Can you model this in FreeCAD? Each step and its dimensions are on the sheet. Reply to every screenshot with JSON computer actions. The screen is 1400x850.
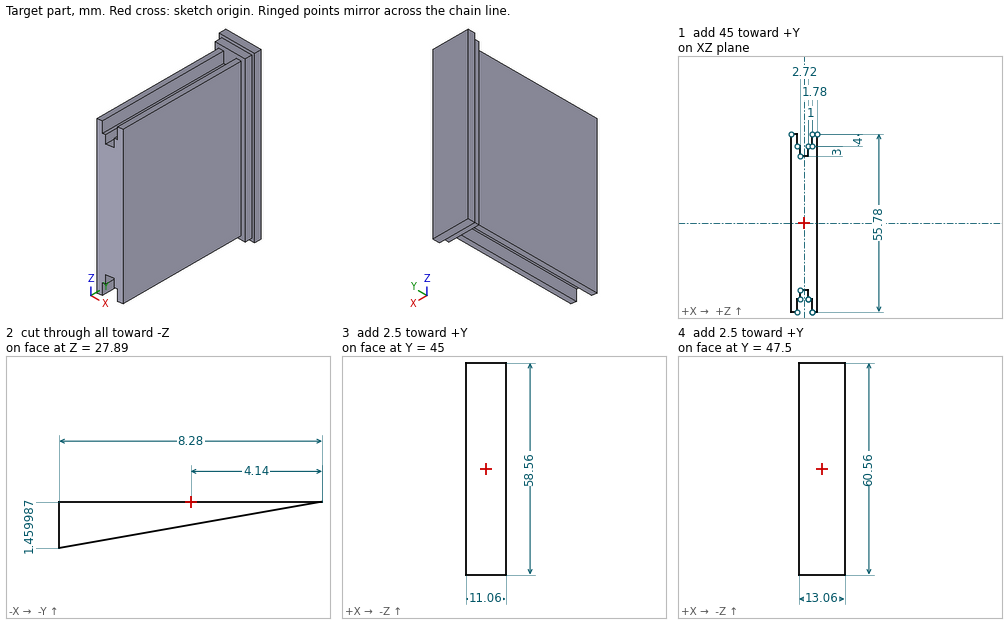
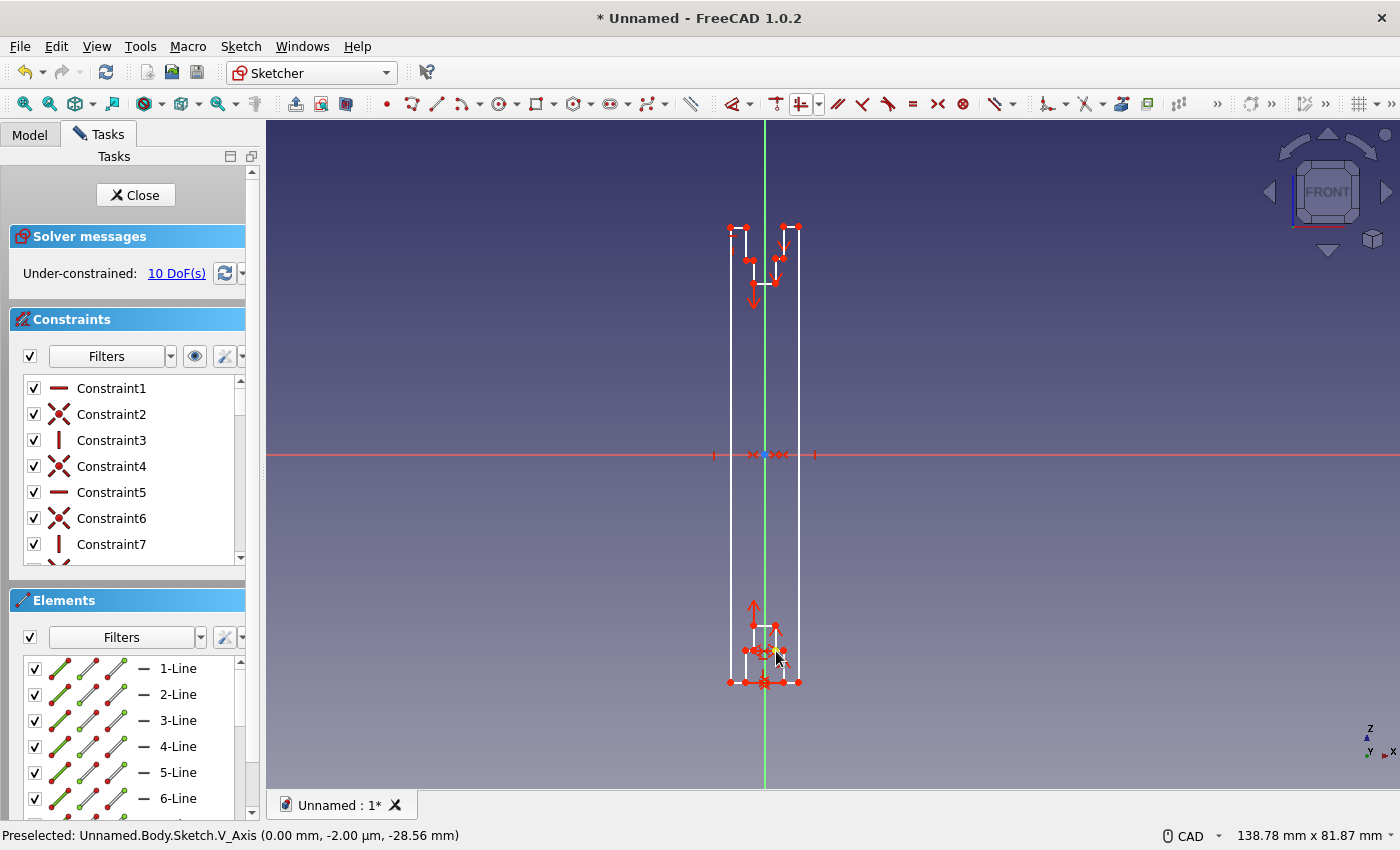
{"action": "left_click", "coordinate": [799, 227]}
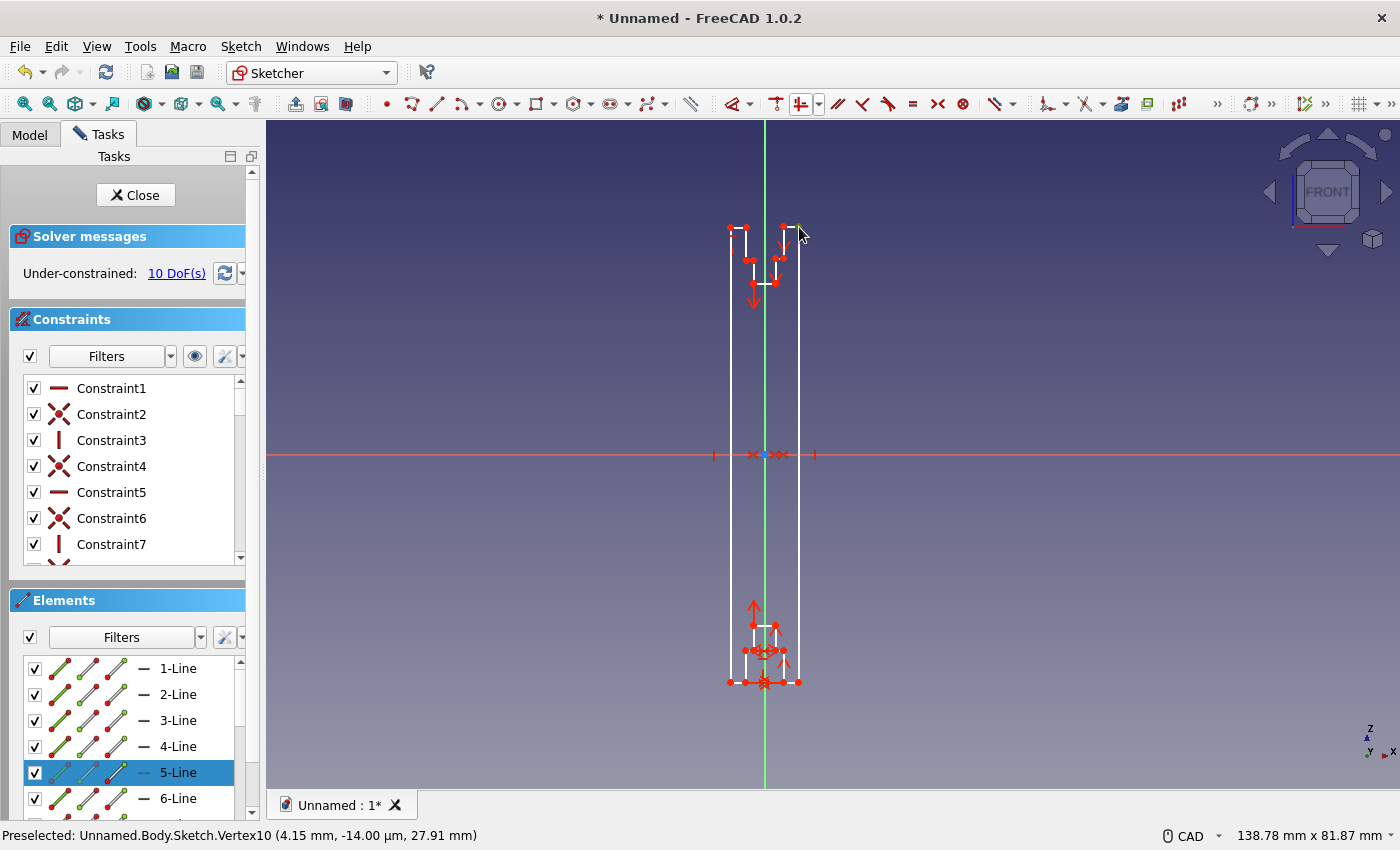
{"action": "left_click", "coordinate": [731, 228]}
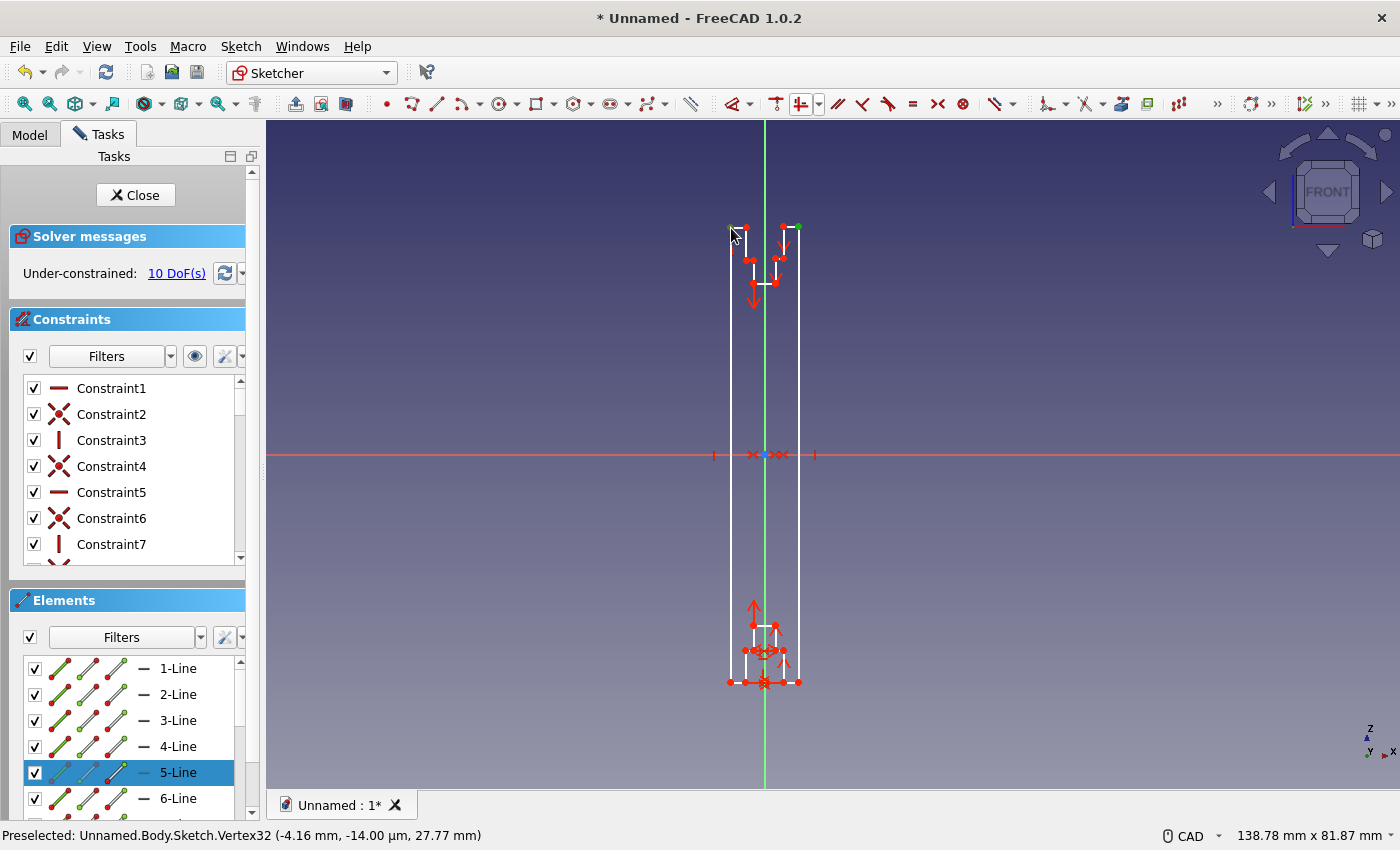
{"action": "left_click", "coordinate": [765, 717]}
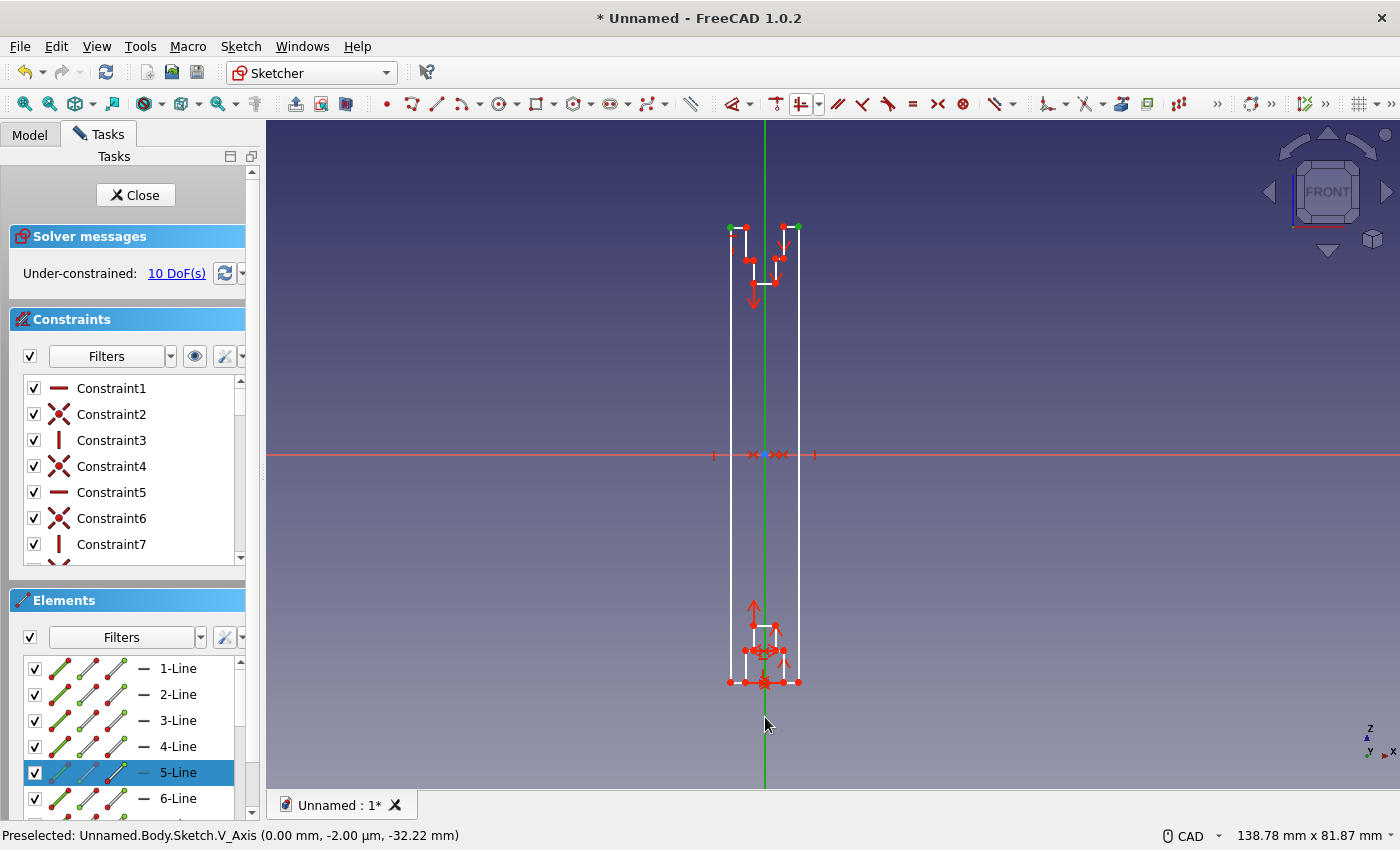
{"action": "left_click", "coordinate": [938, 104]}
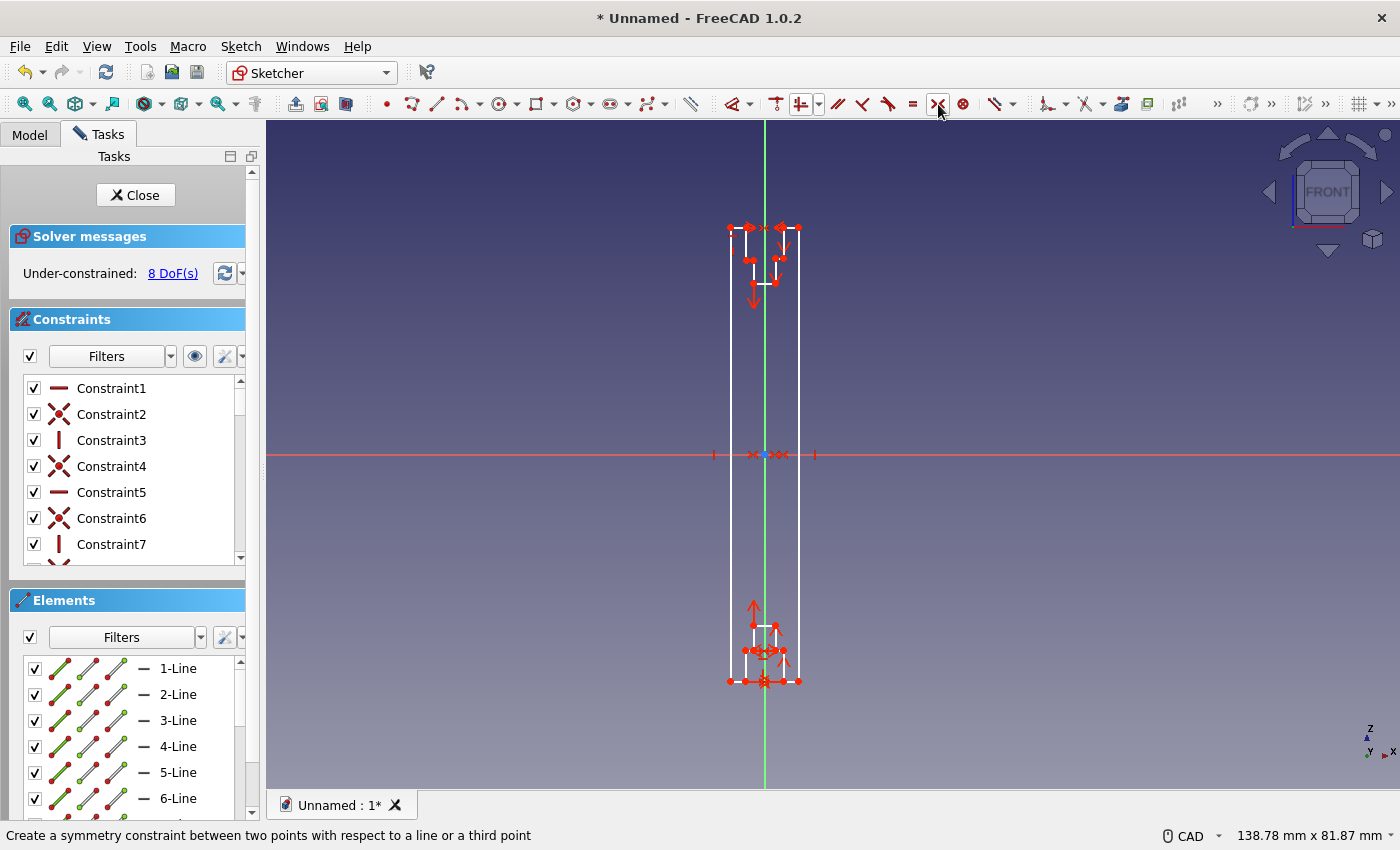
{"action": "scroll", "coordinate": [784, 259], "scroll_direction": "up", "scroll_amount": 3}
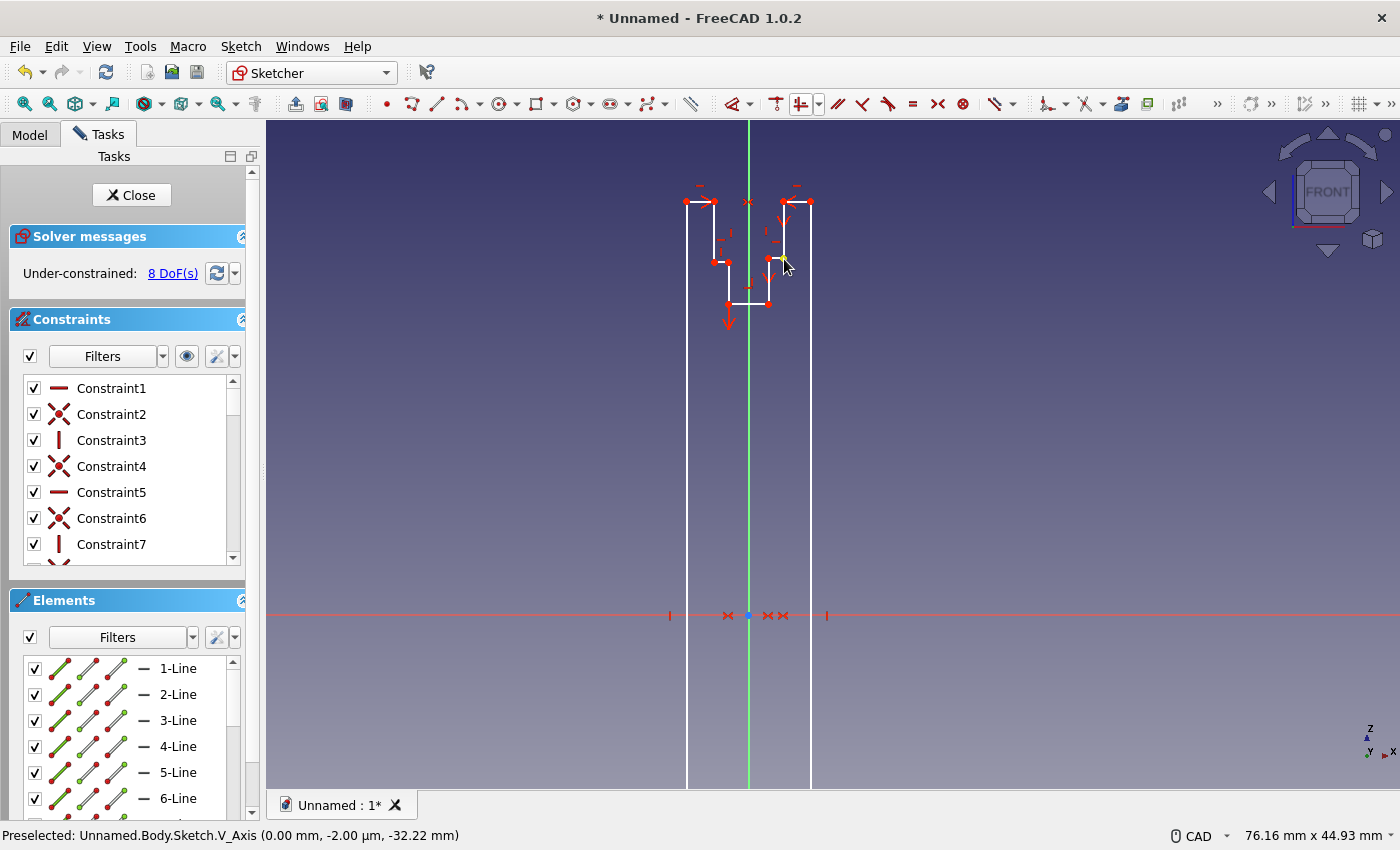
{"action": "left_click", "coordinate": [784, 258]}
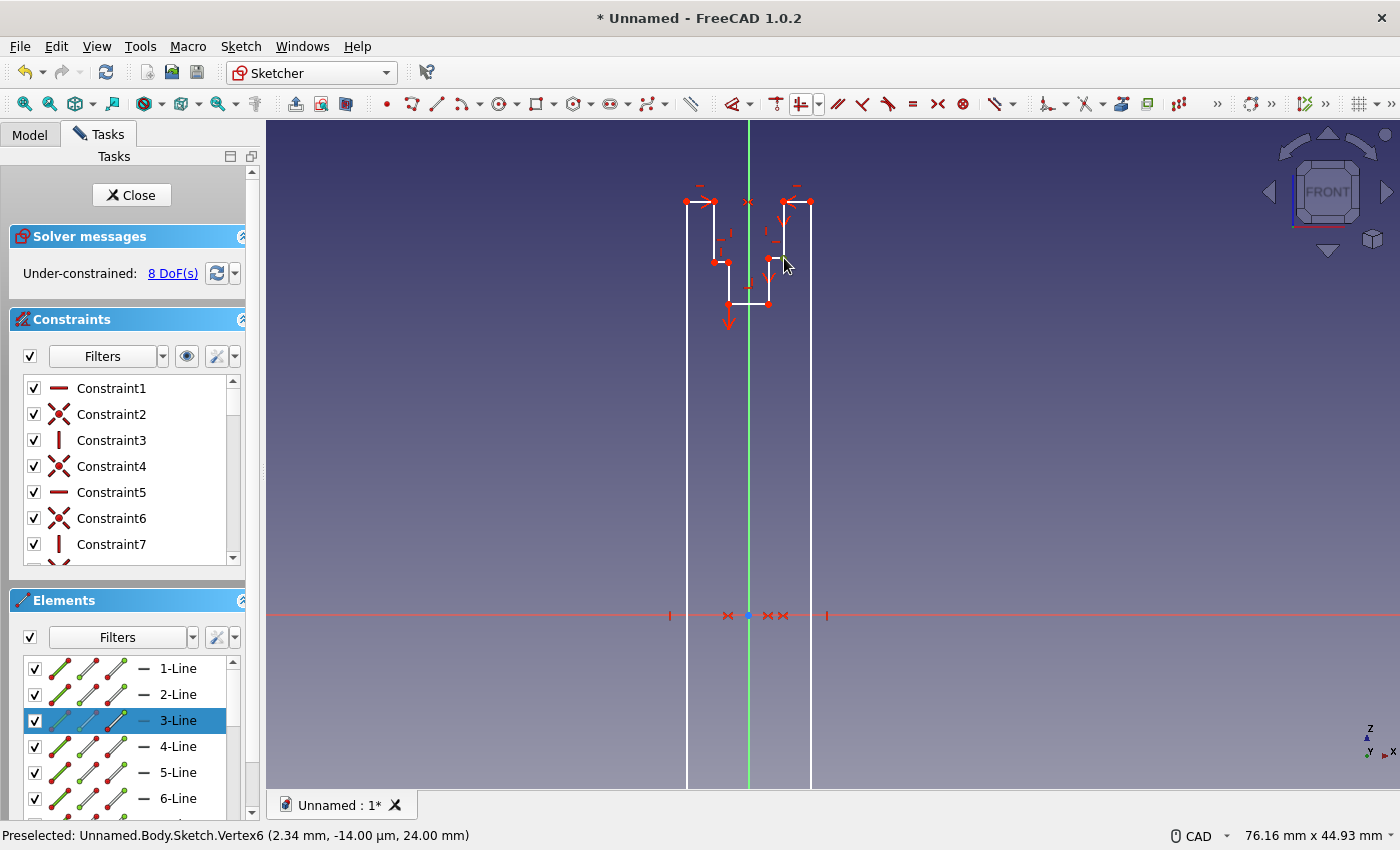
{"action": "left_click", "coordinate": [714, 262]}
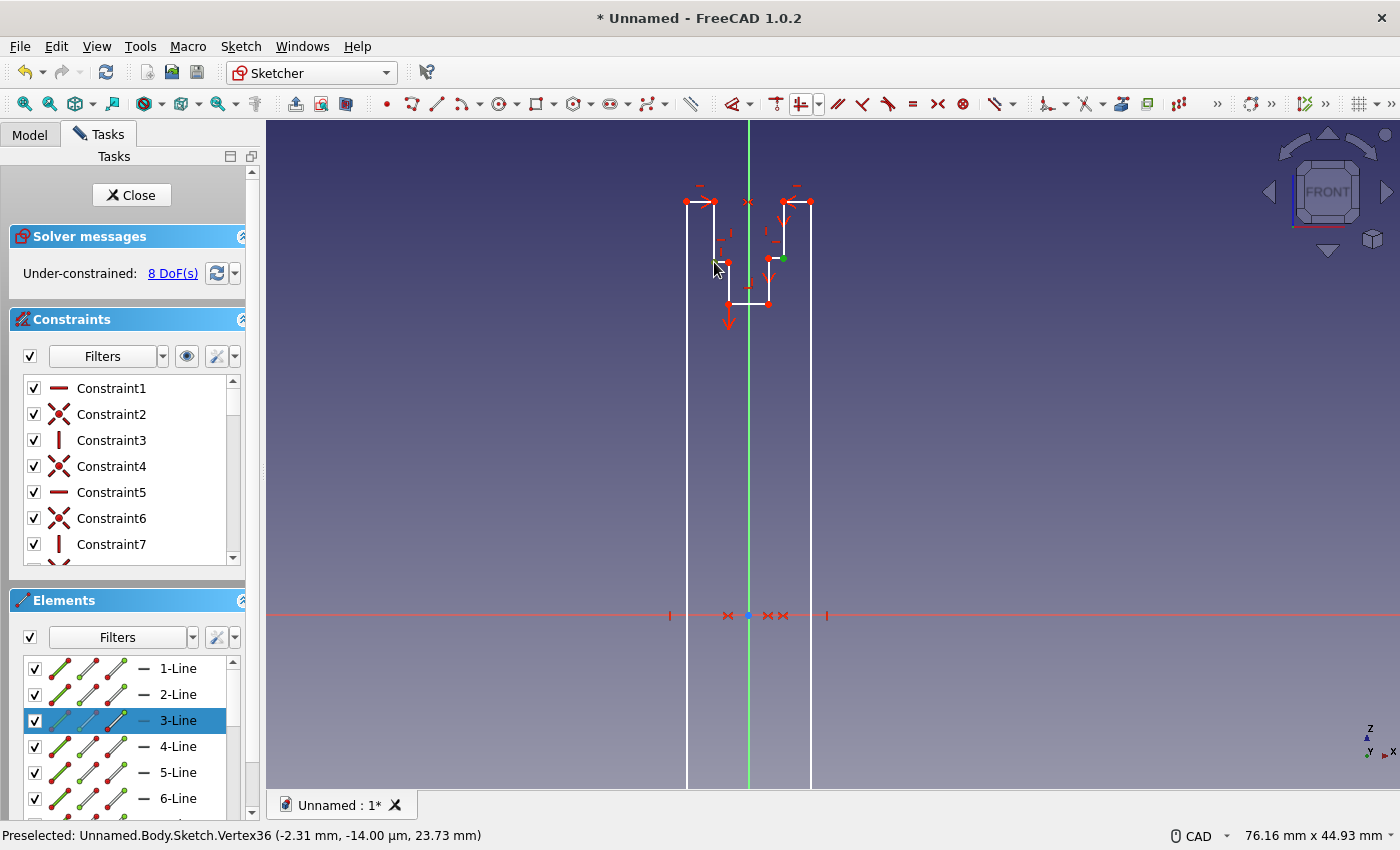
{"action": "left_click", "coordinate": [749, 717]}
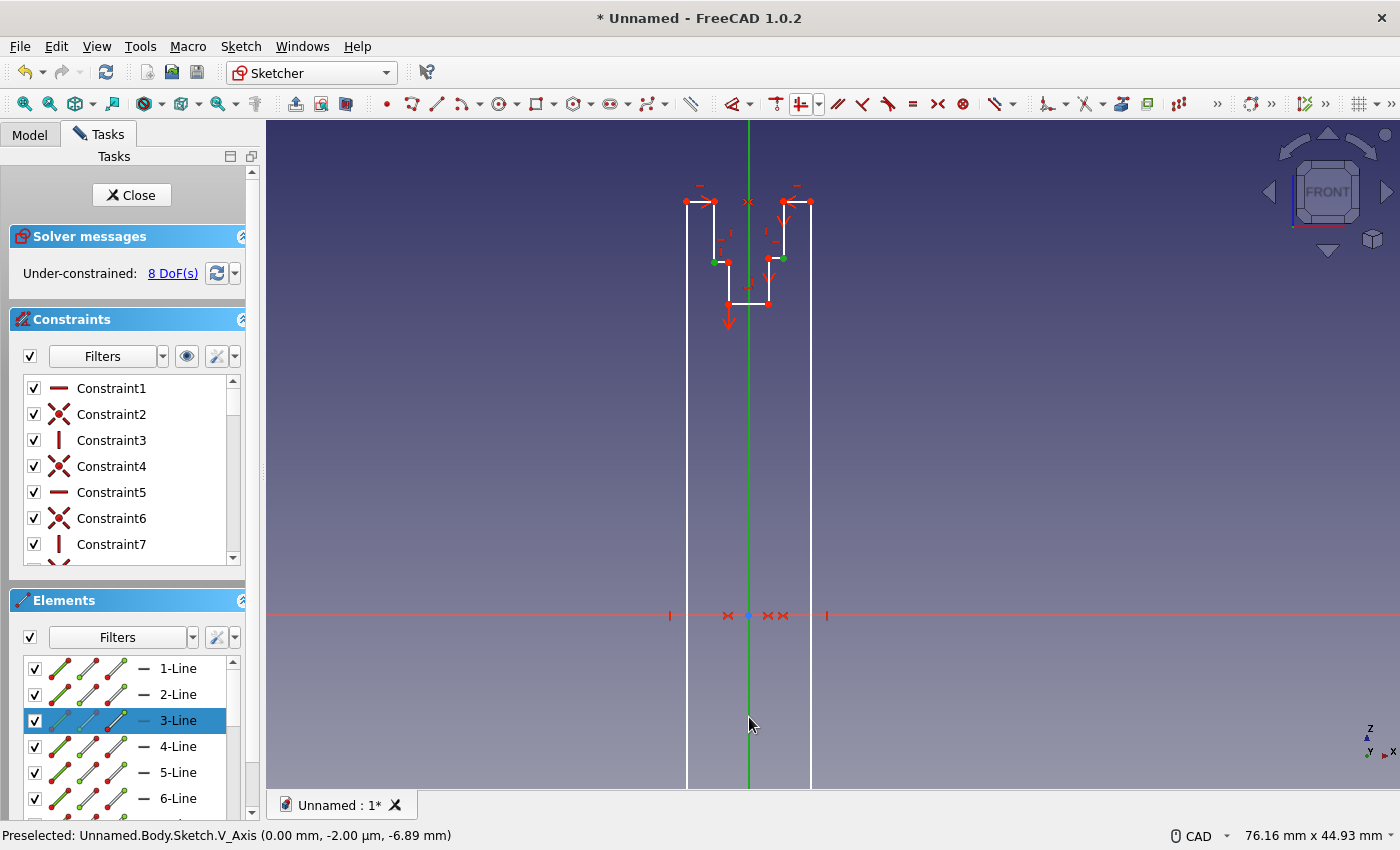
{"action": "left_click", "coordinate": [938, 104]}